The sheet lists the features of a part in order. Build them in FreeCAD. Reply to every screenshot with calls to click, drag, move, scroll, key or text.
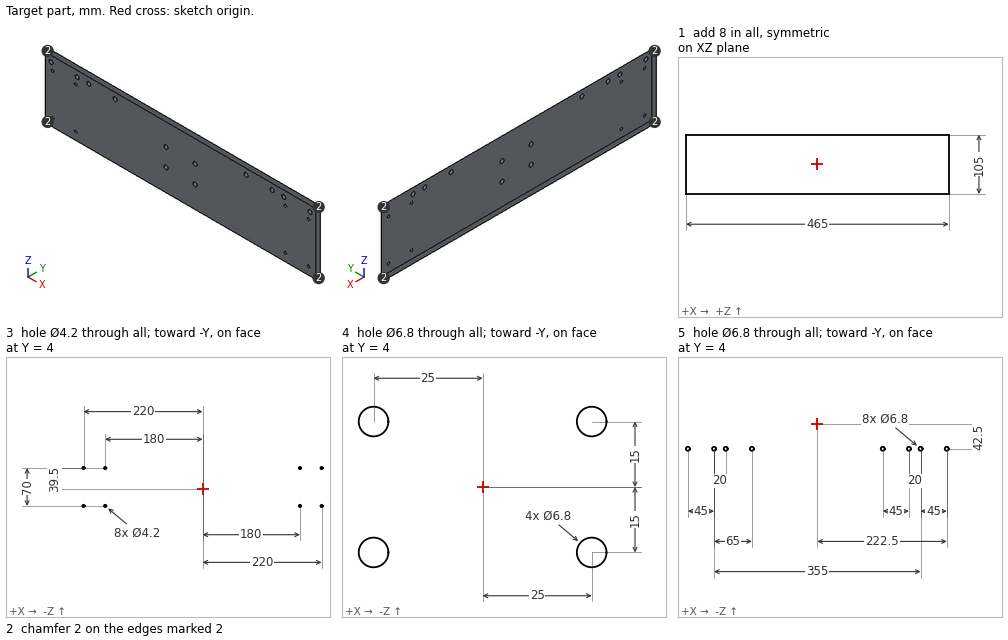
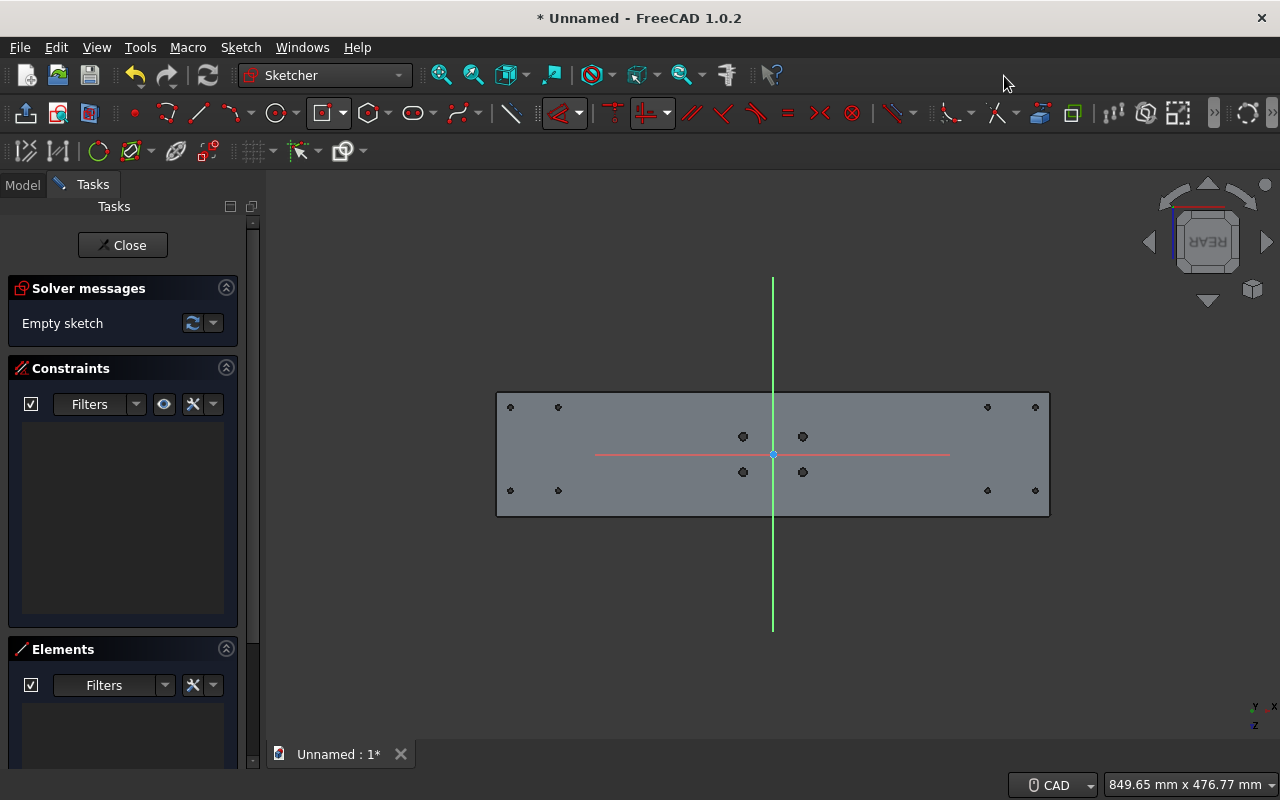
click(276, 114)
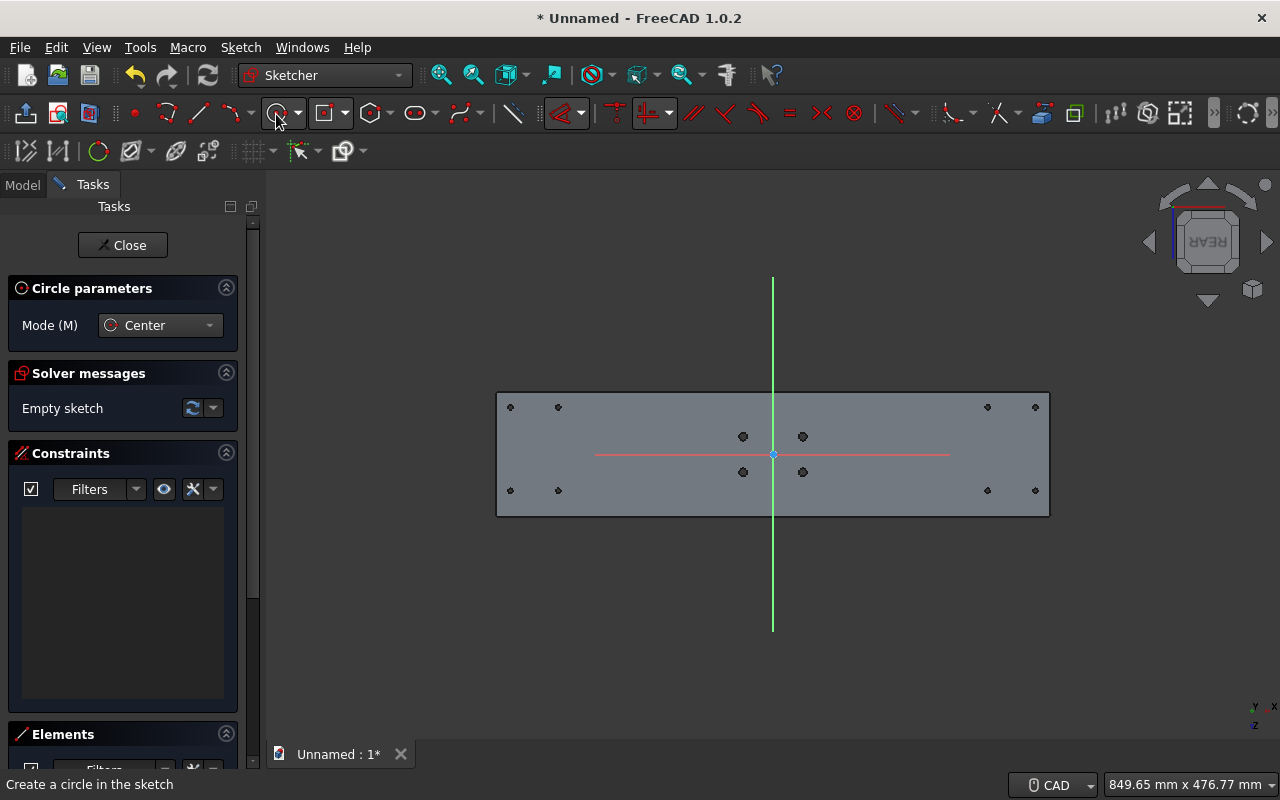
scroll(1039, 505, up, 9)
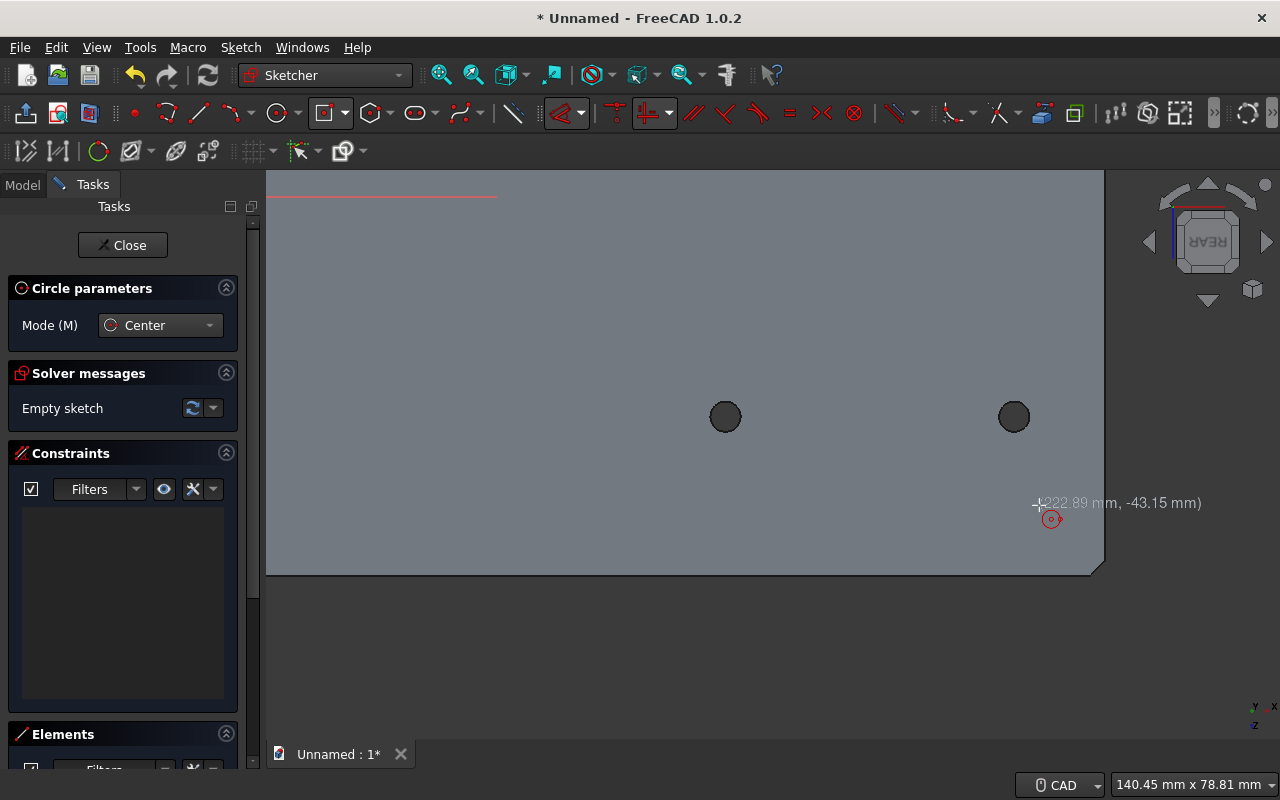
scroll(958, 473, down, 9)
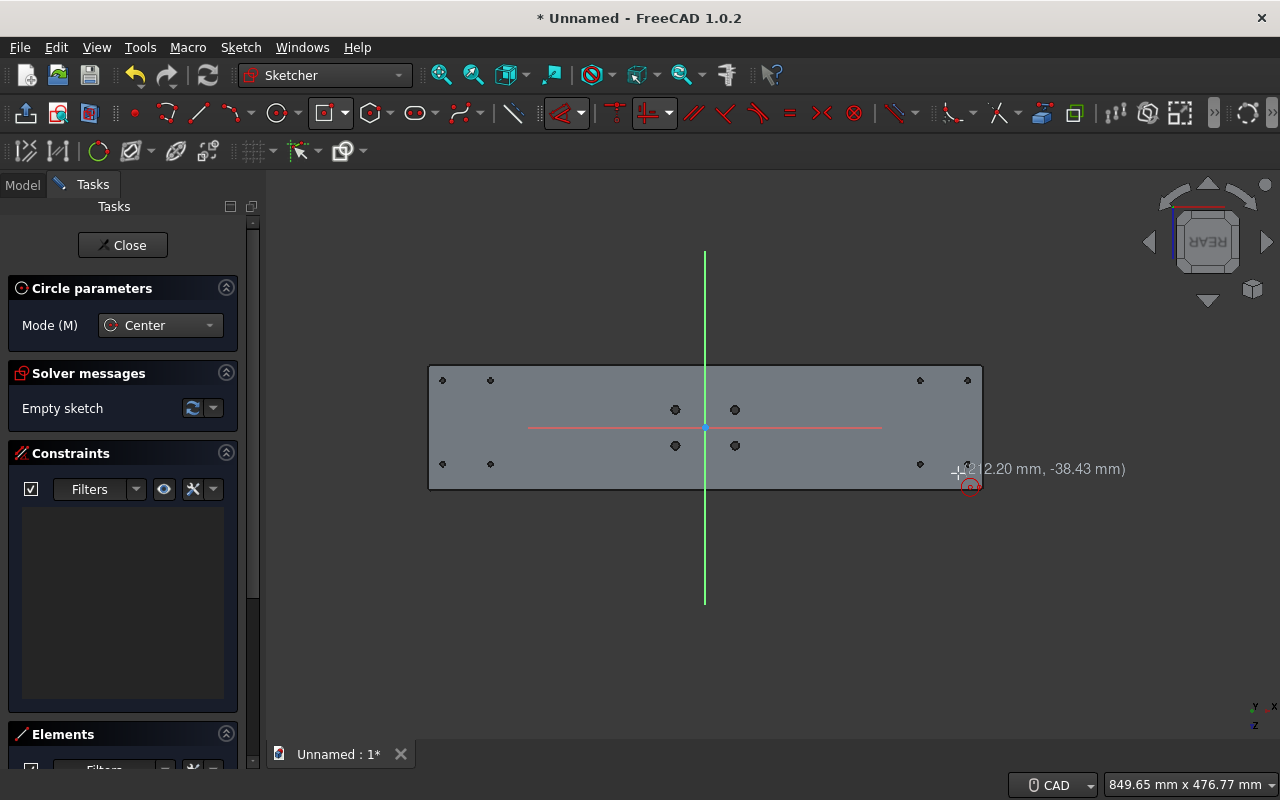
click(971, 478)
move(974, 476)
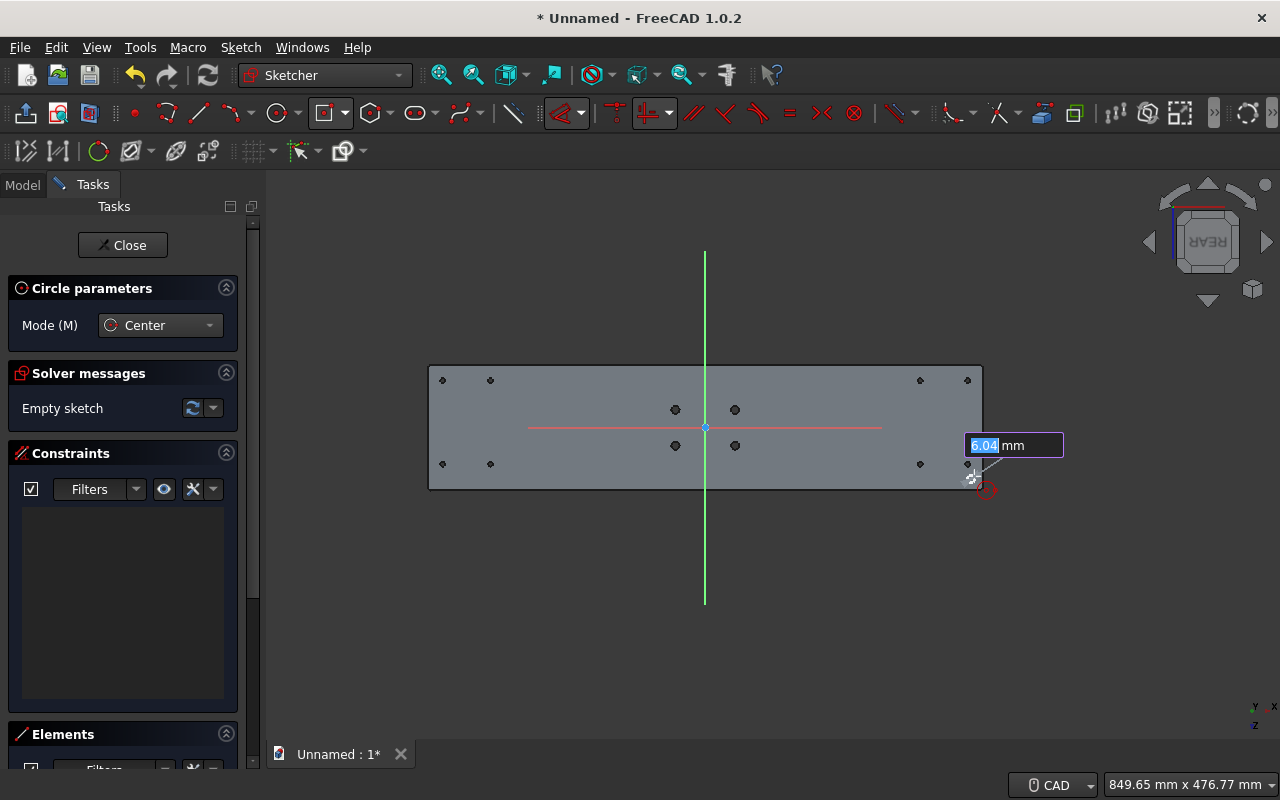
text(6.8)
key(Return)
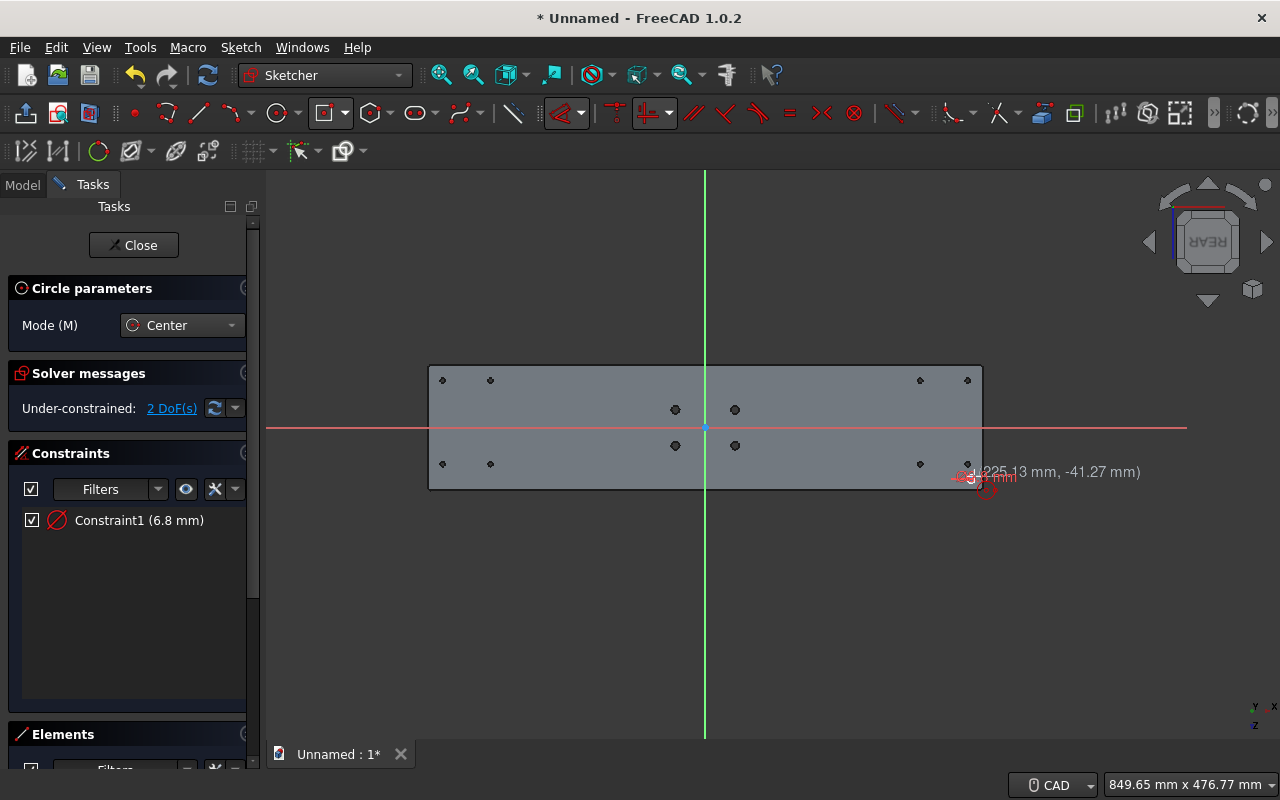
scroll(917, 478, up, 9)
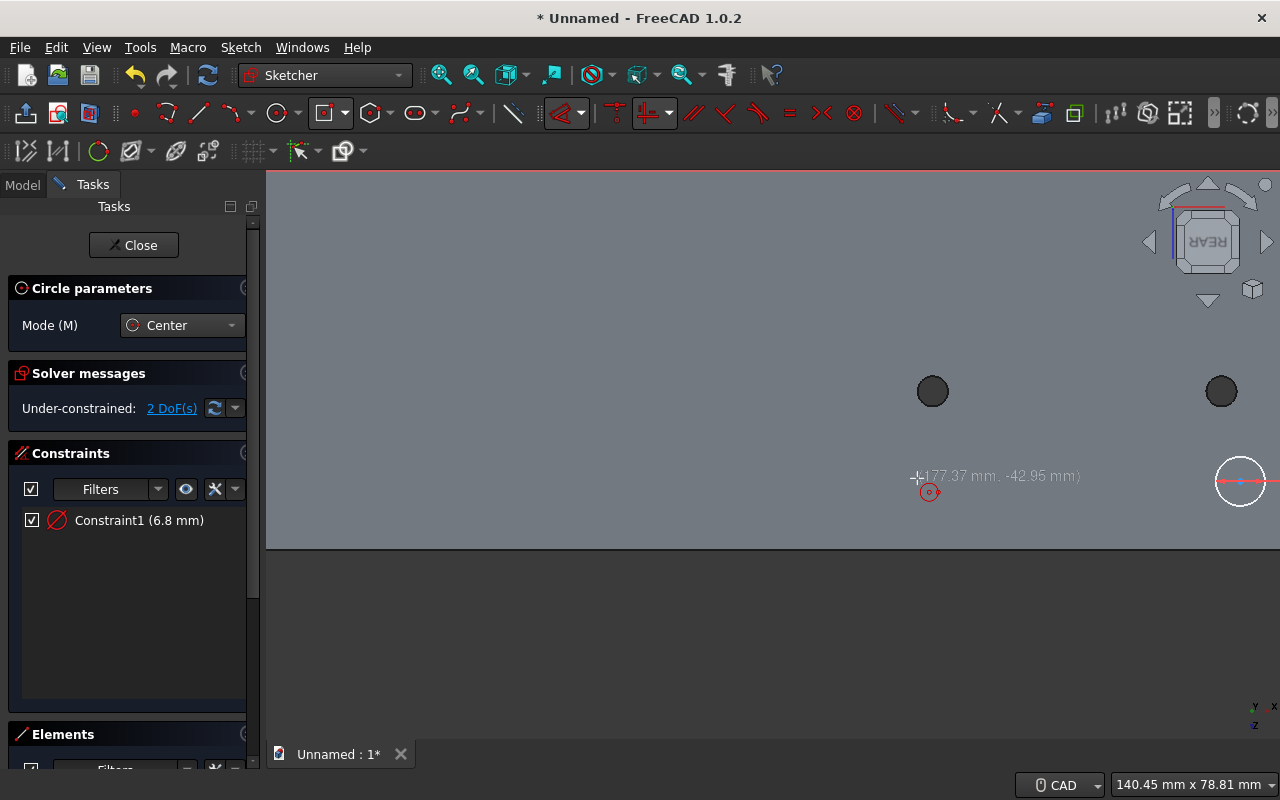
scroll(917, 478, down, 9)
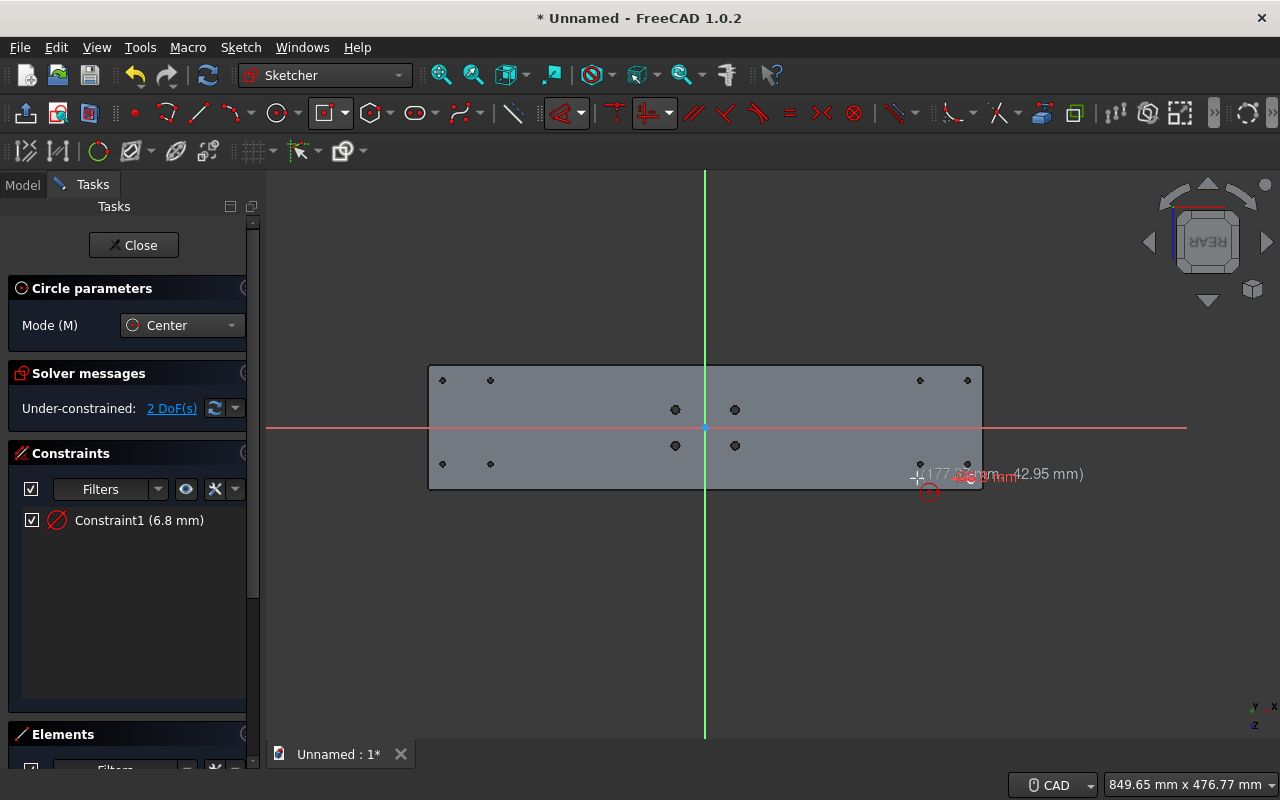
click(917, 478)
move(920, 476)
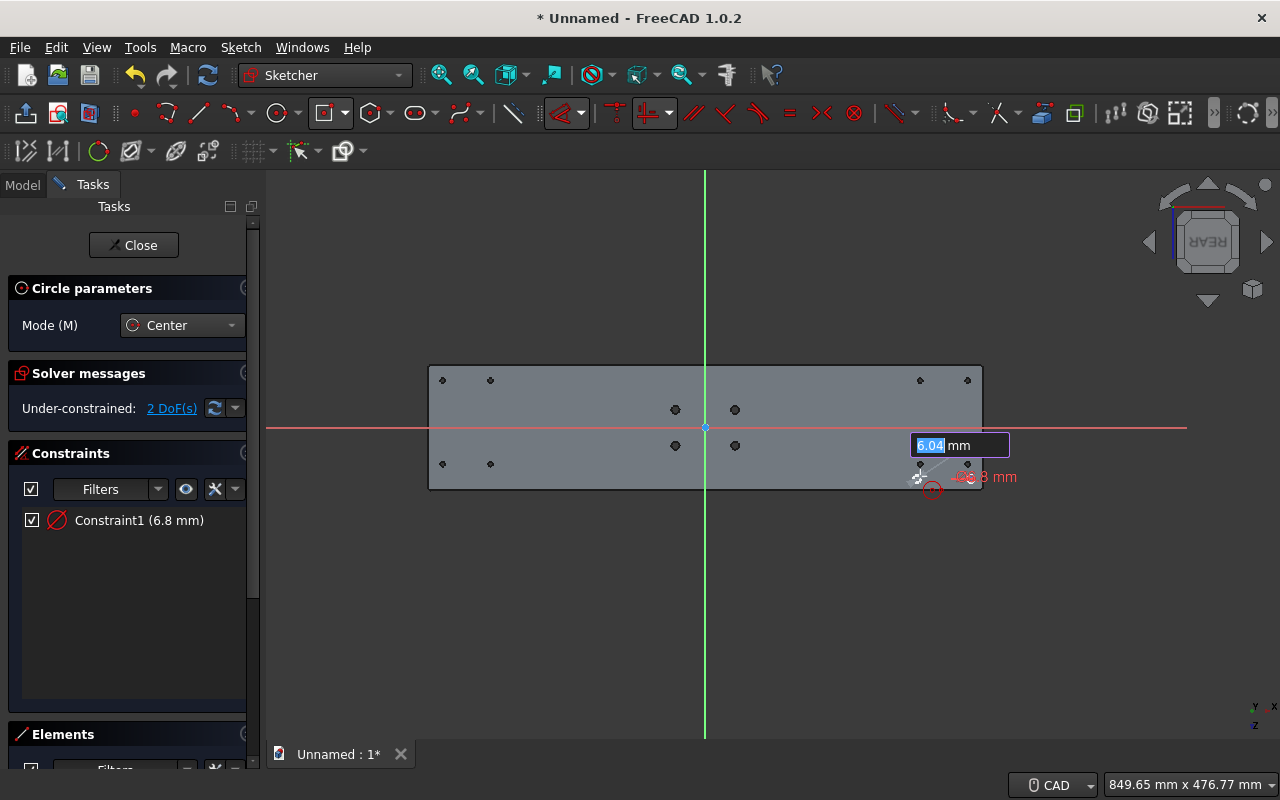
text(6.8)
key(Return)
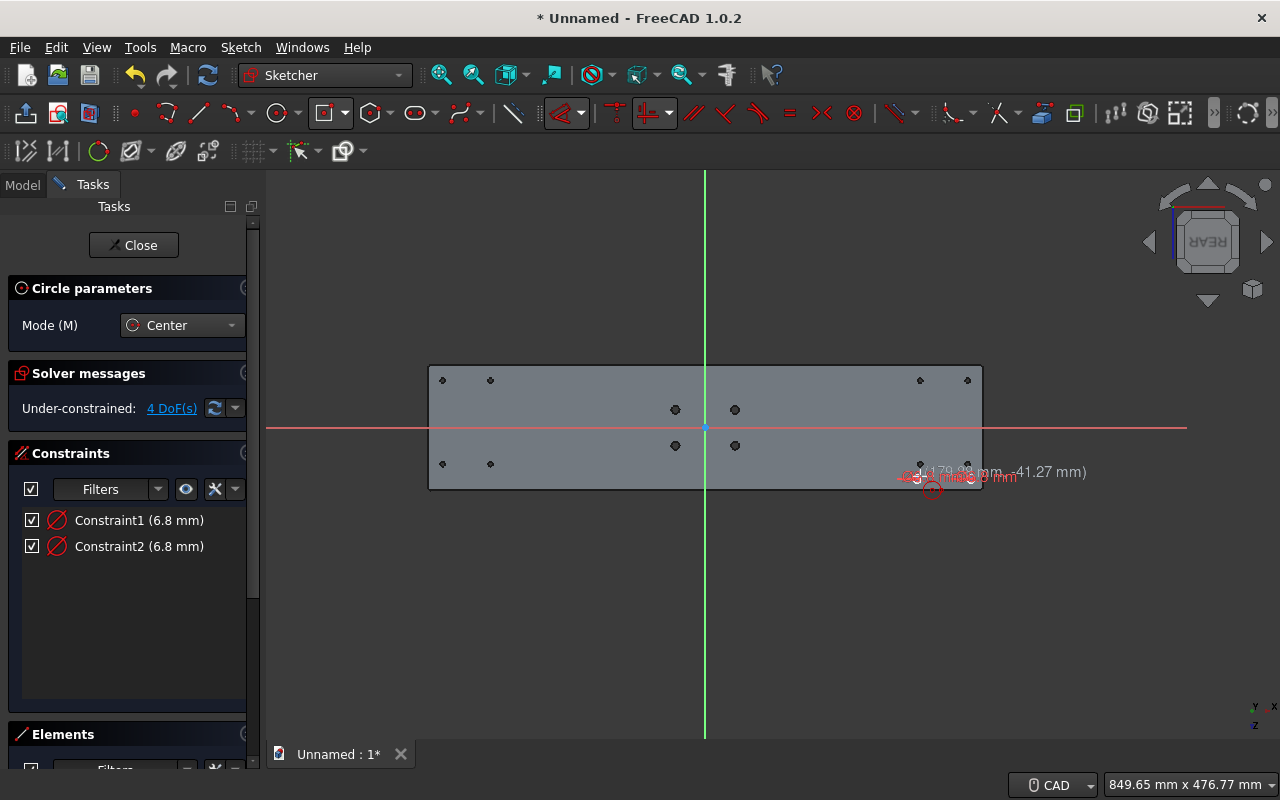
scroll(493, 478, up, 9)